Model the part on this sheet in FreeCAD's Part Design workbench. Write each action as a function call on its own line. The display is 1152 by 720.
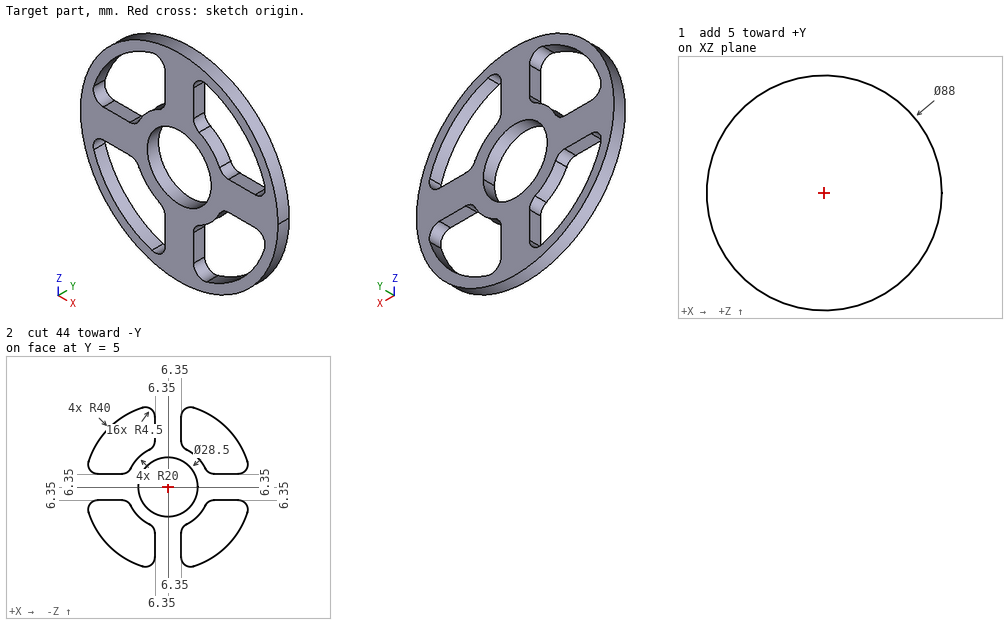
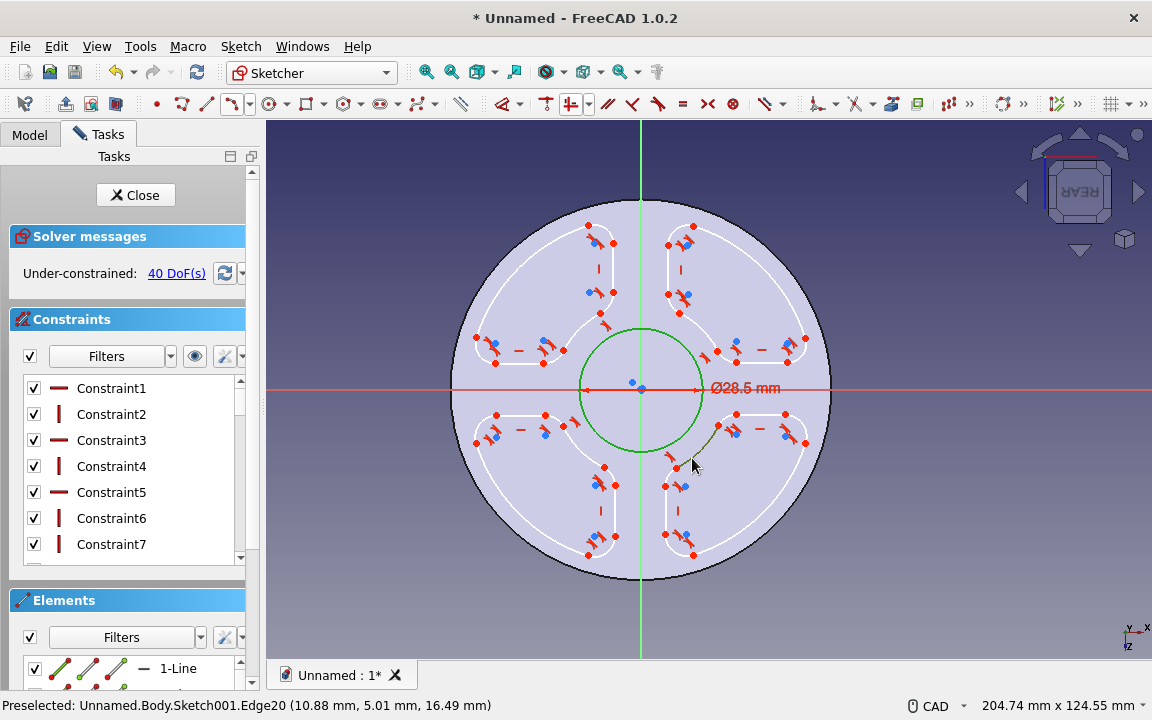
click(546, 104)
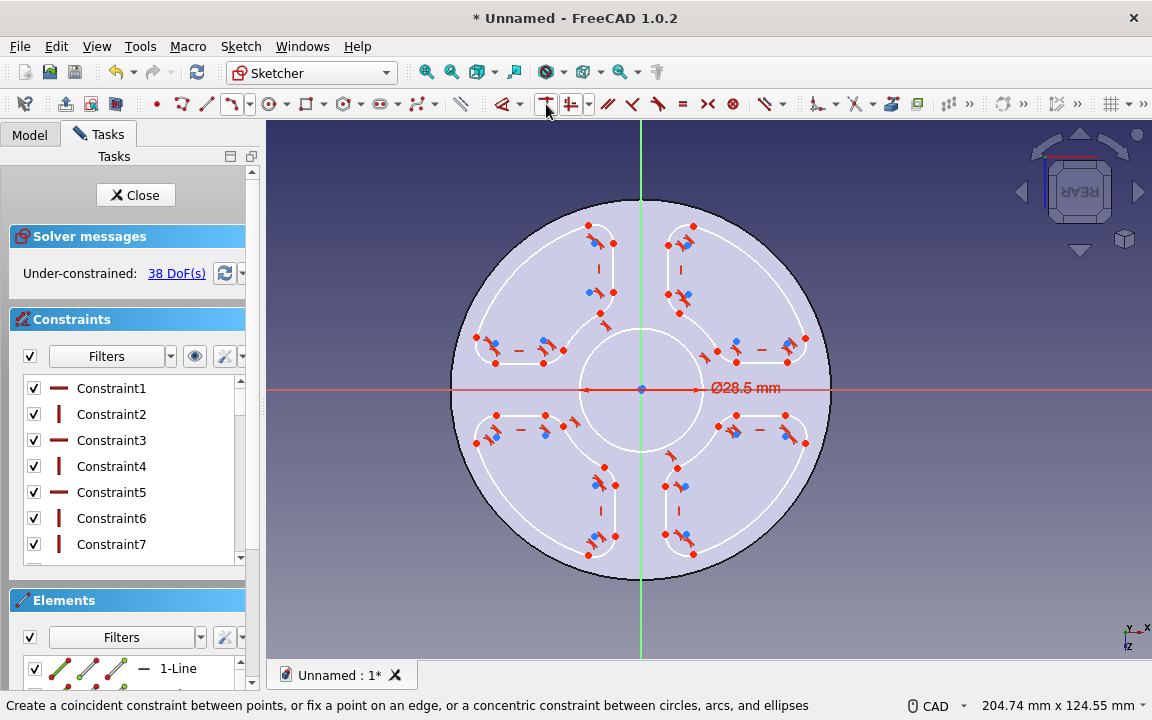
click(685, 346)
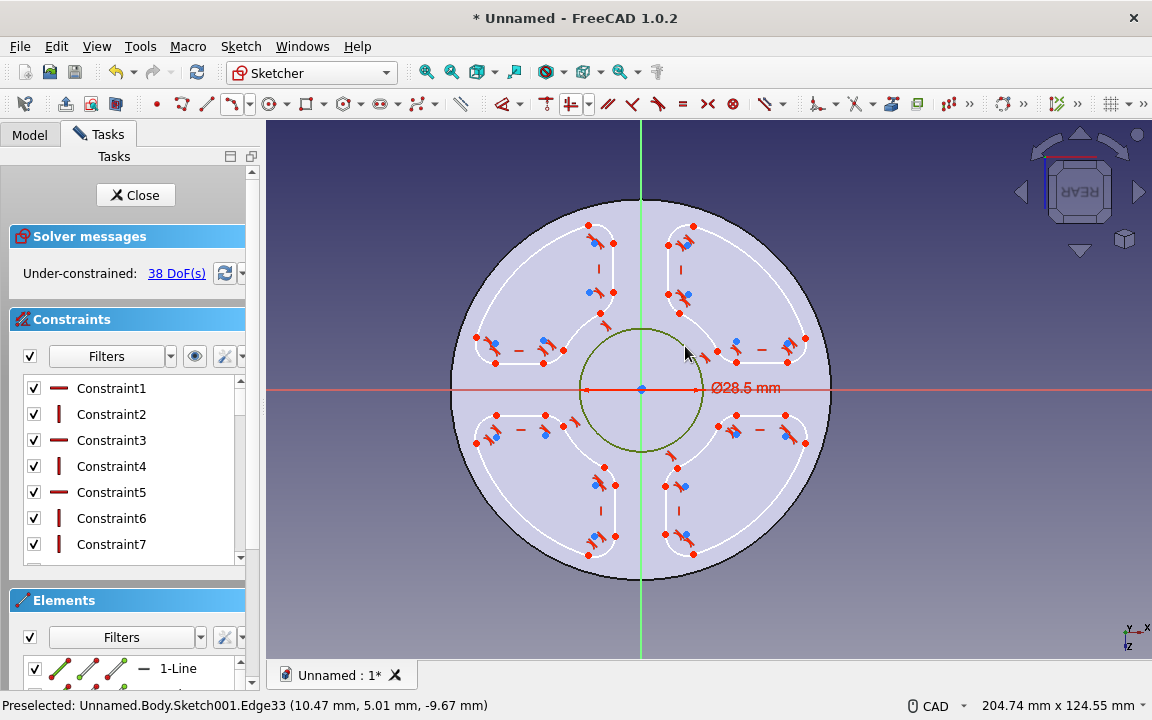
click(573, 442)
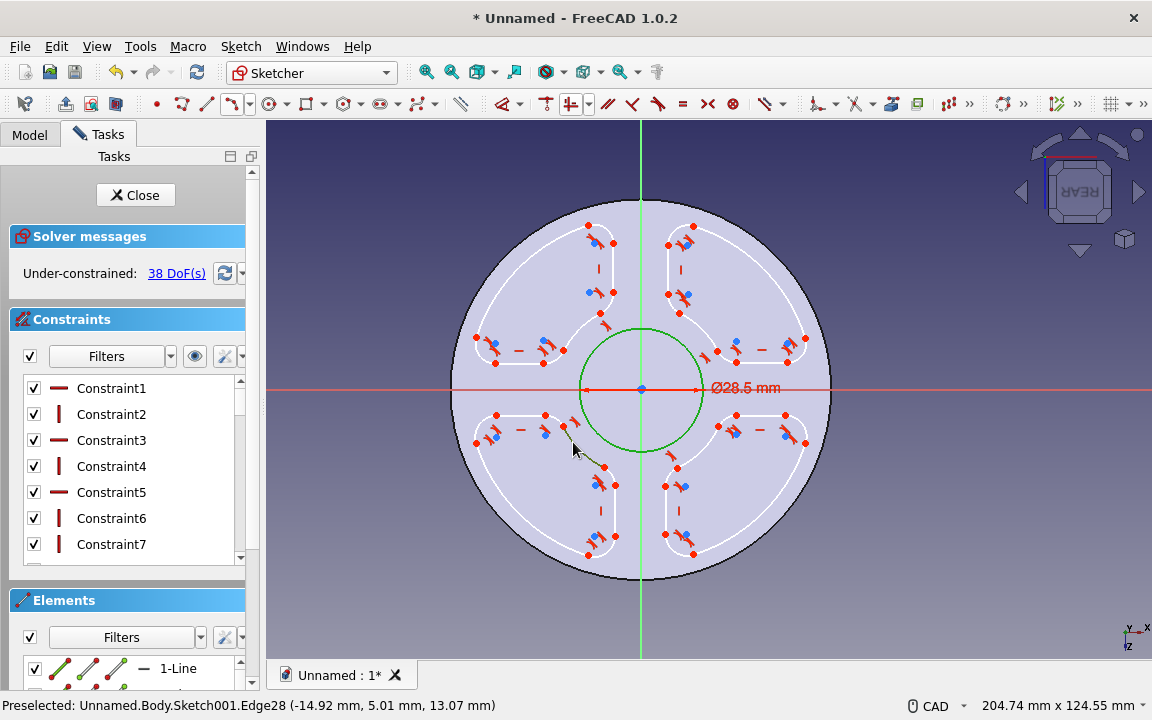
click(546, 104)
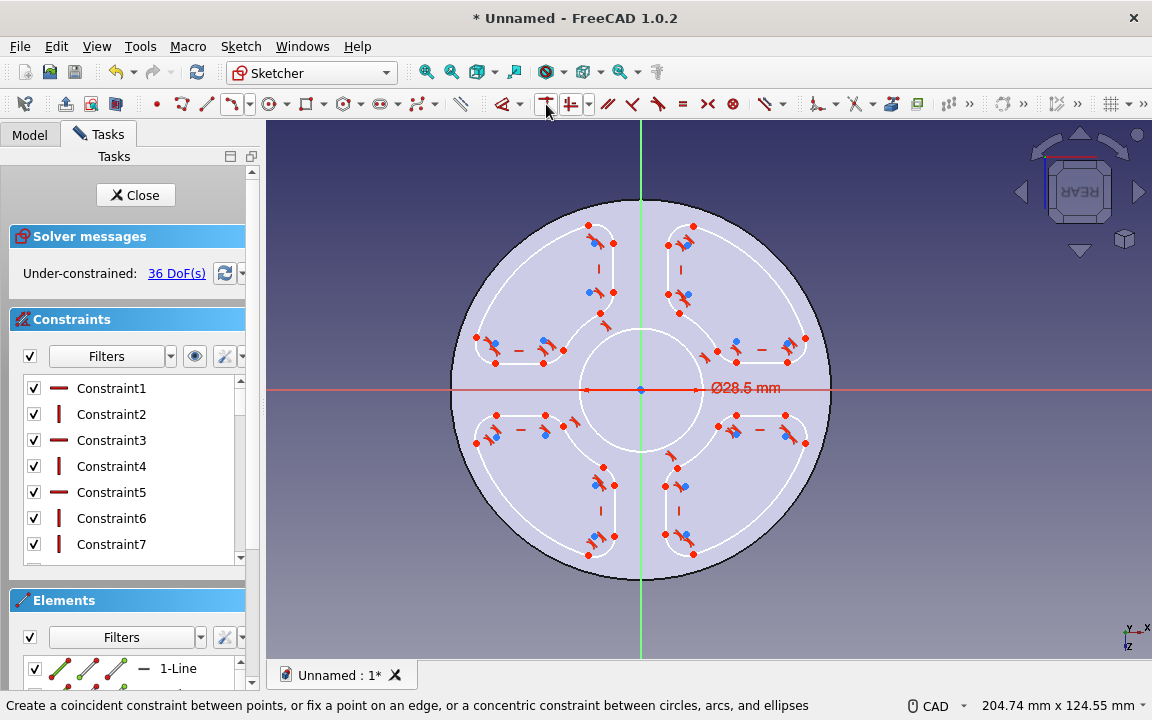
click(685, 346)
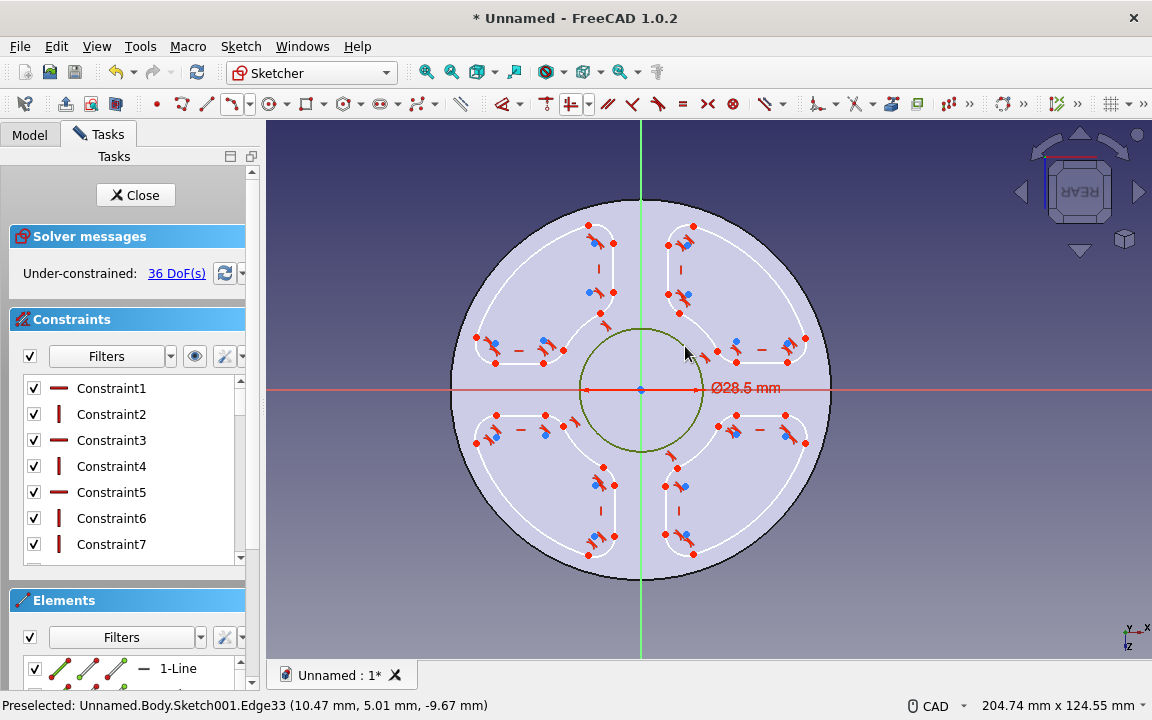
click(498, 488)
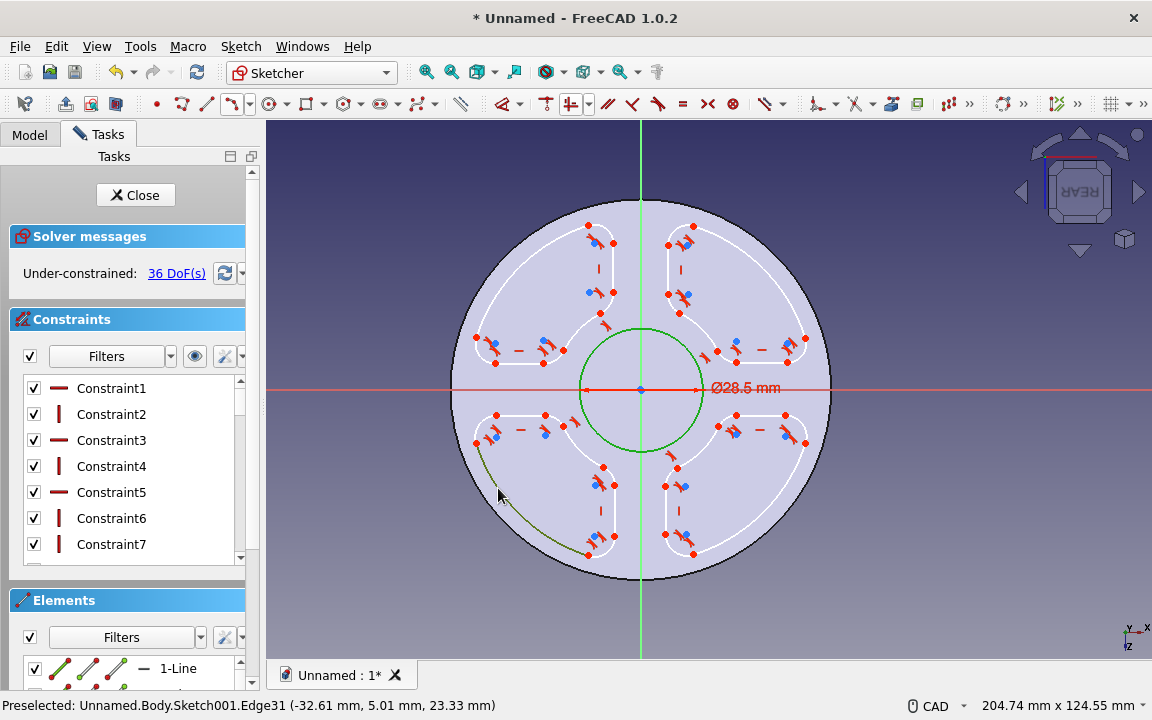
key(c)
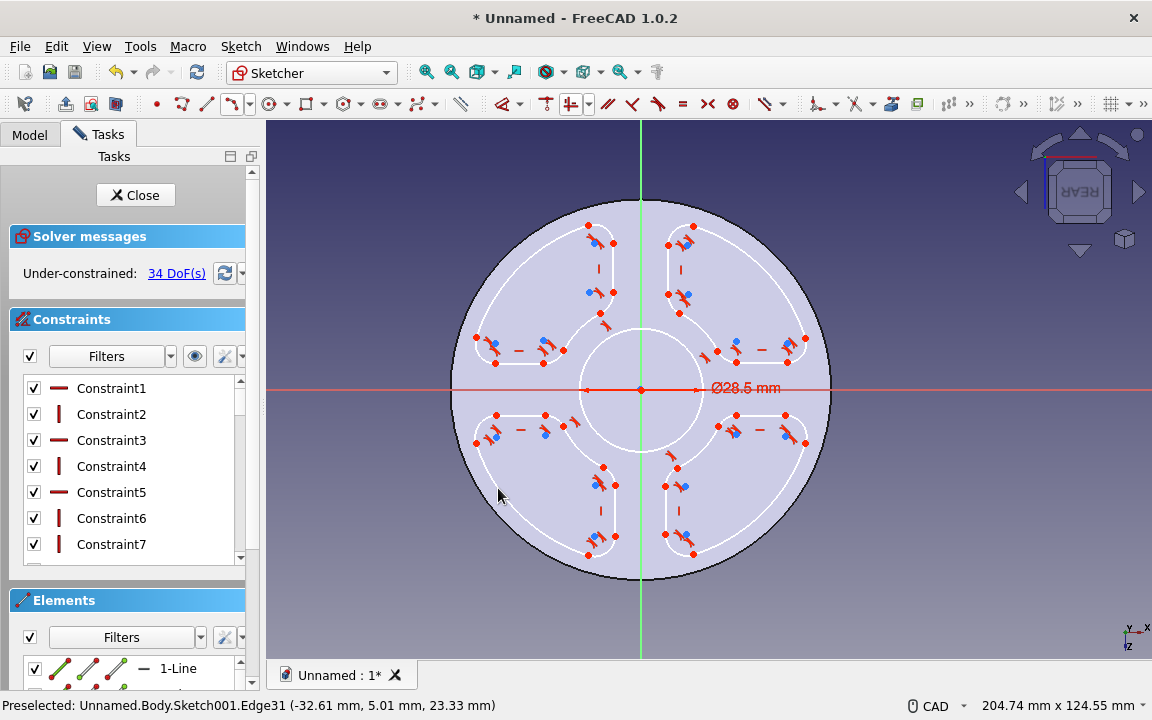
scroll(641, 390, up, 4)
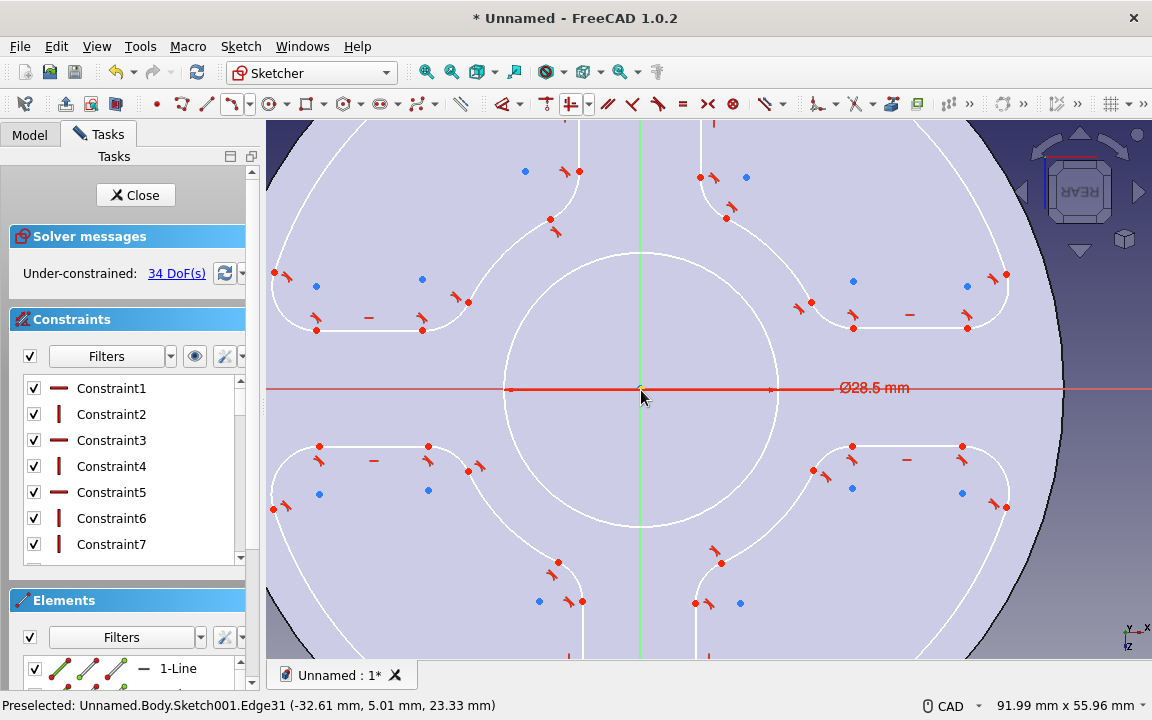
drag(630, 379, 651, 400)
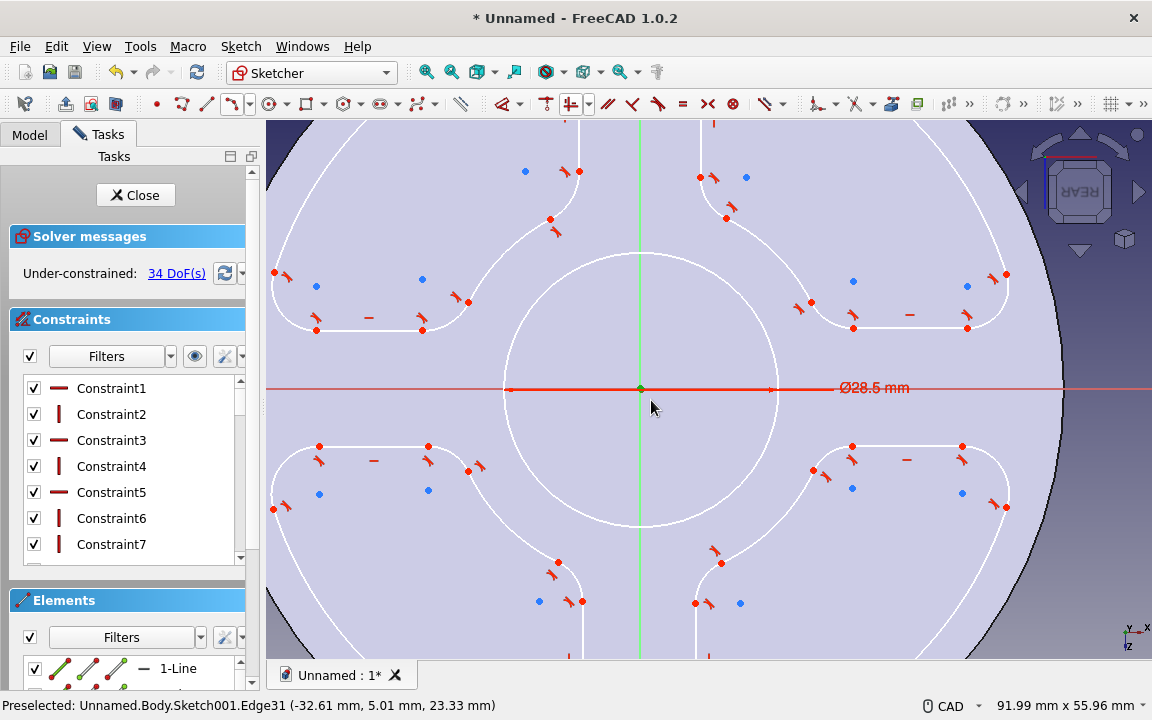
click(546, 104)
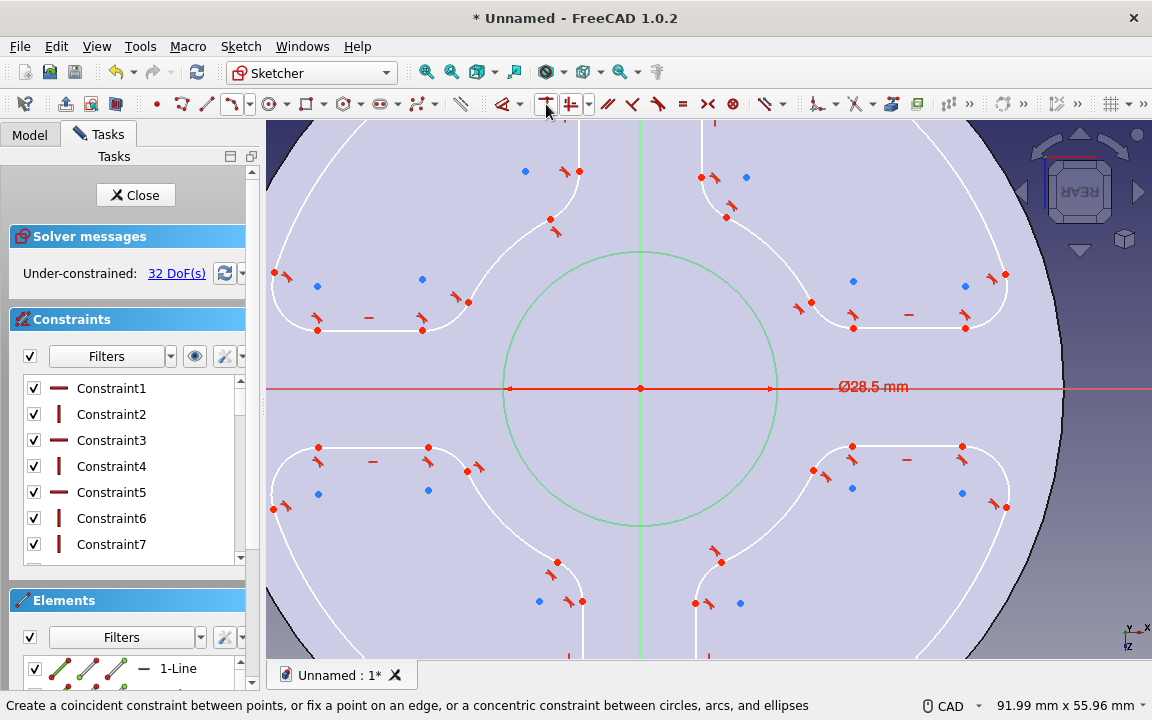
click(440, 328)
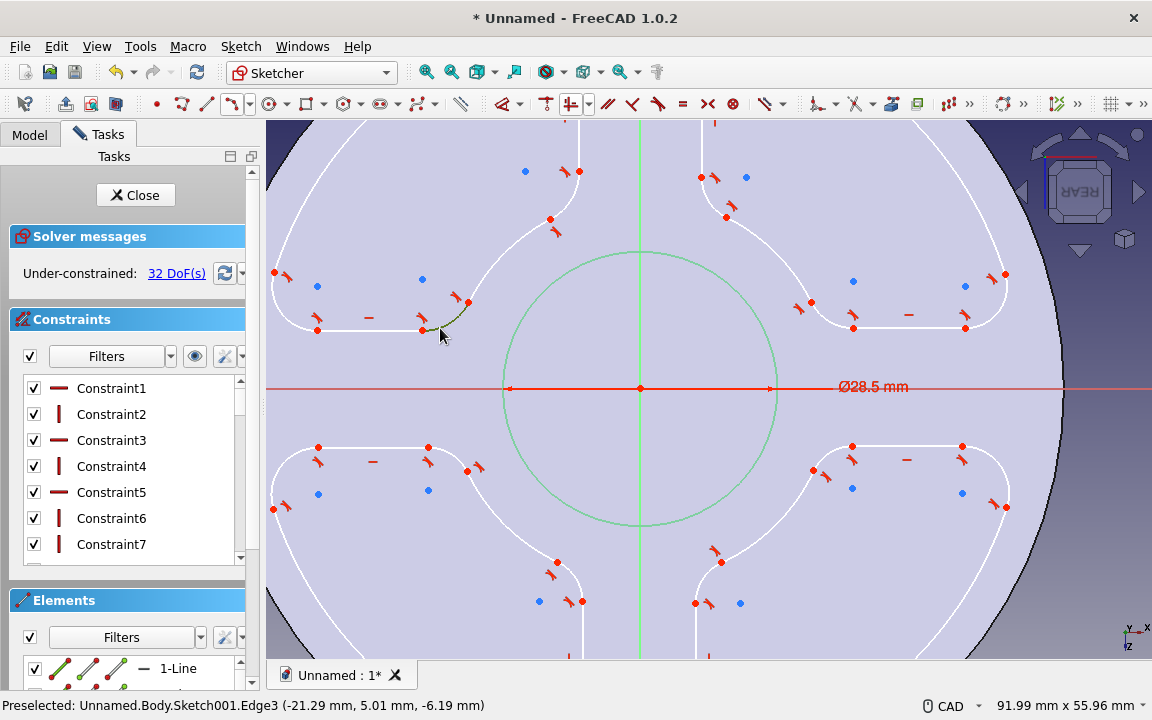
click(564, 209)